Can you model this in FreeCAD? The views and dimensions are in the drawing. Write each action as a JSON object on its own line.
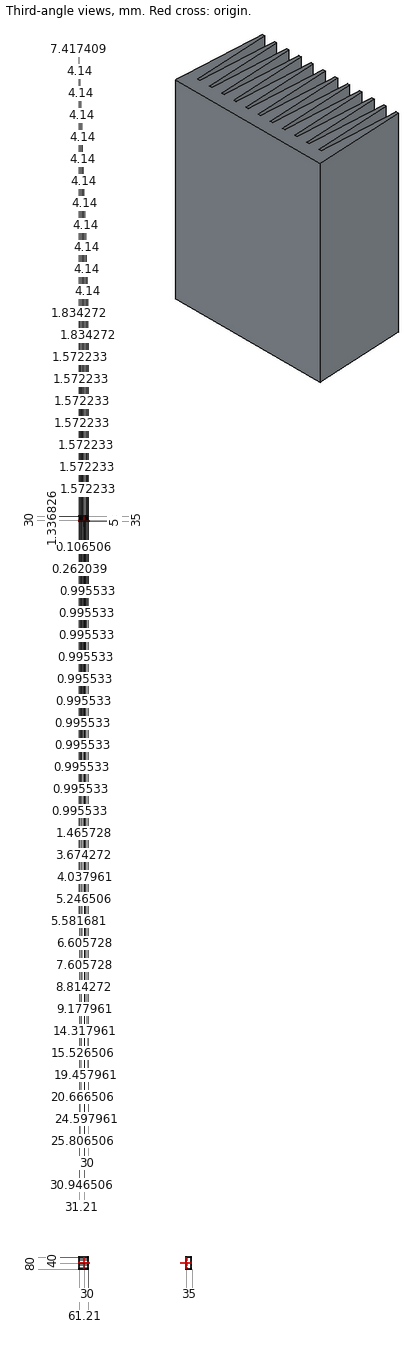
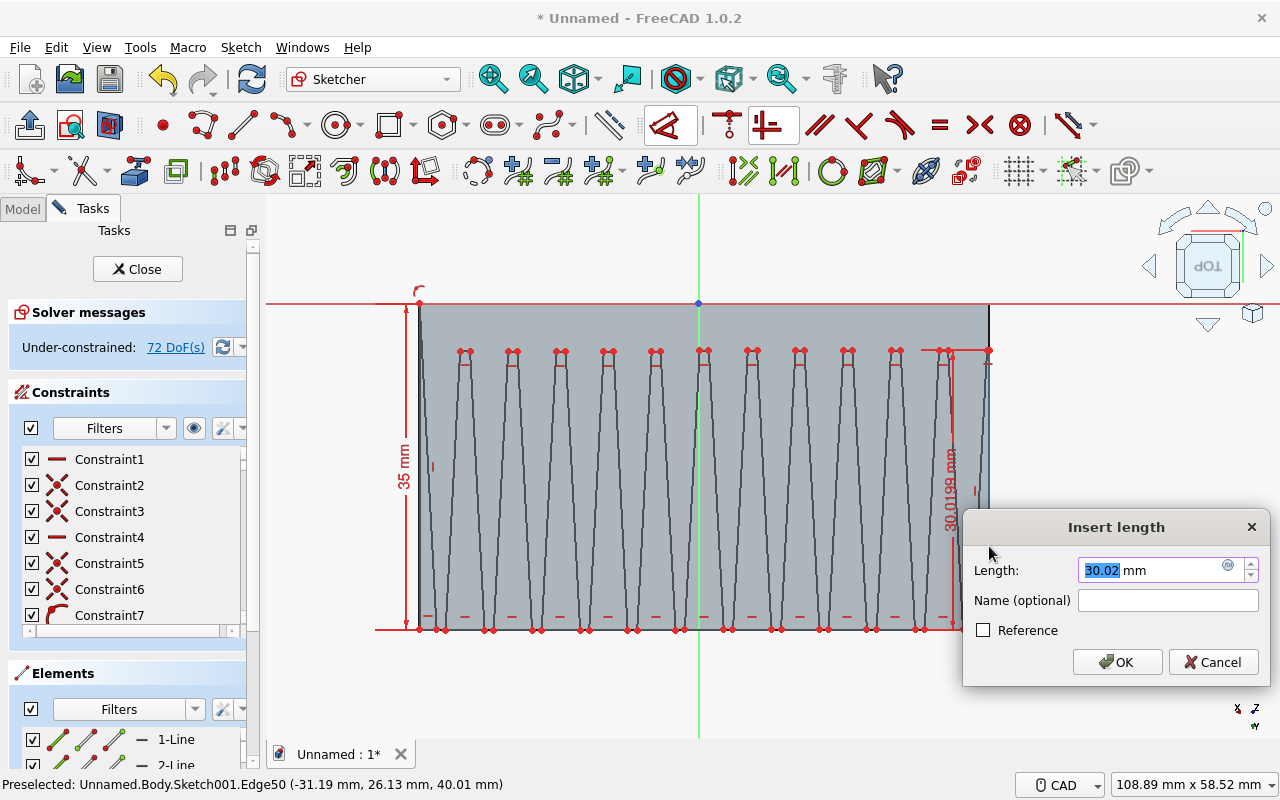
{"action": "type", "text": "30"}
{"action": "key", "text": "Return"}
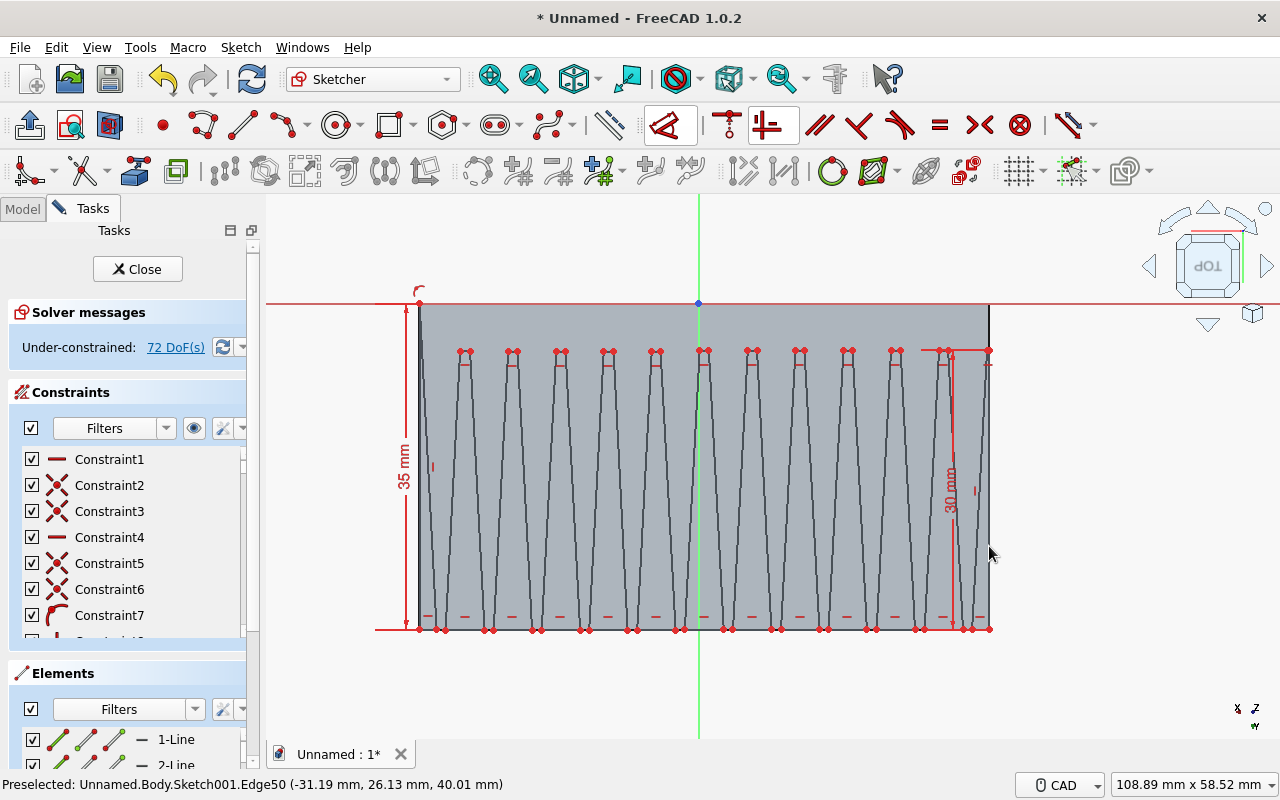
{"action": "scroll", "coordinate": [470, 351], "scroll_direction": "up", "scroll_amount": 2}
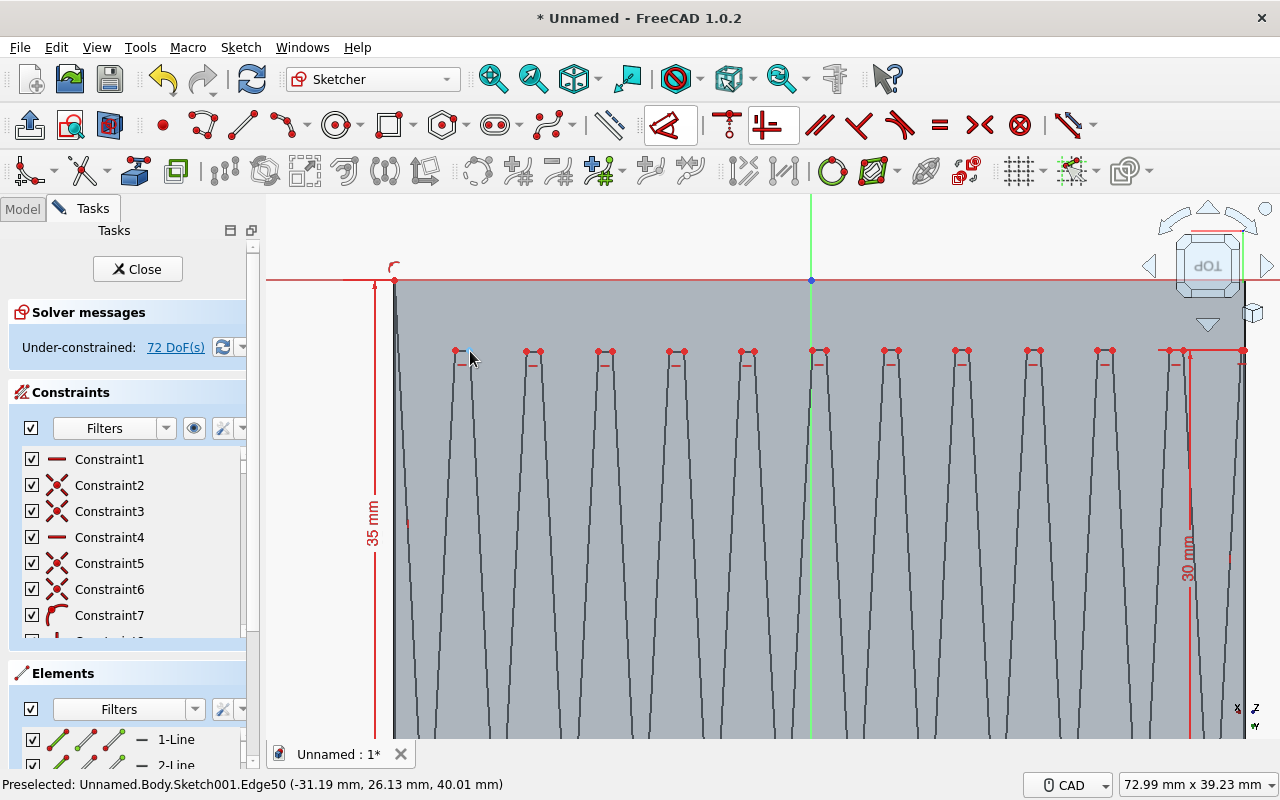
{"action": "left_click", "coordinate": [470, 351]}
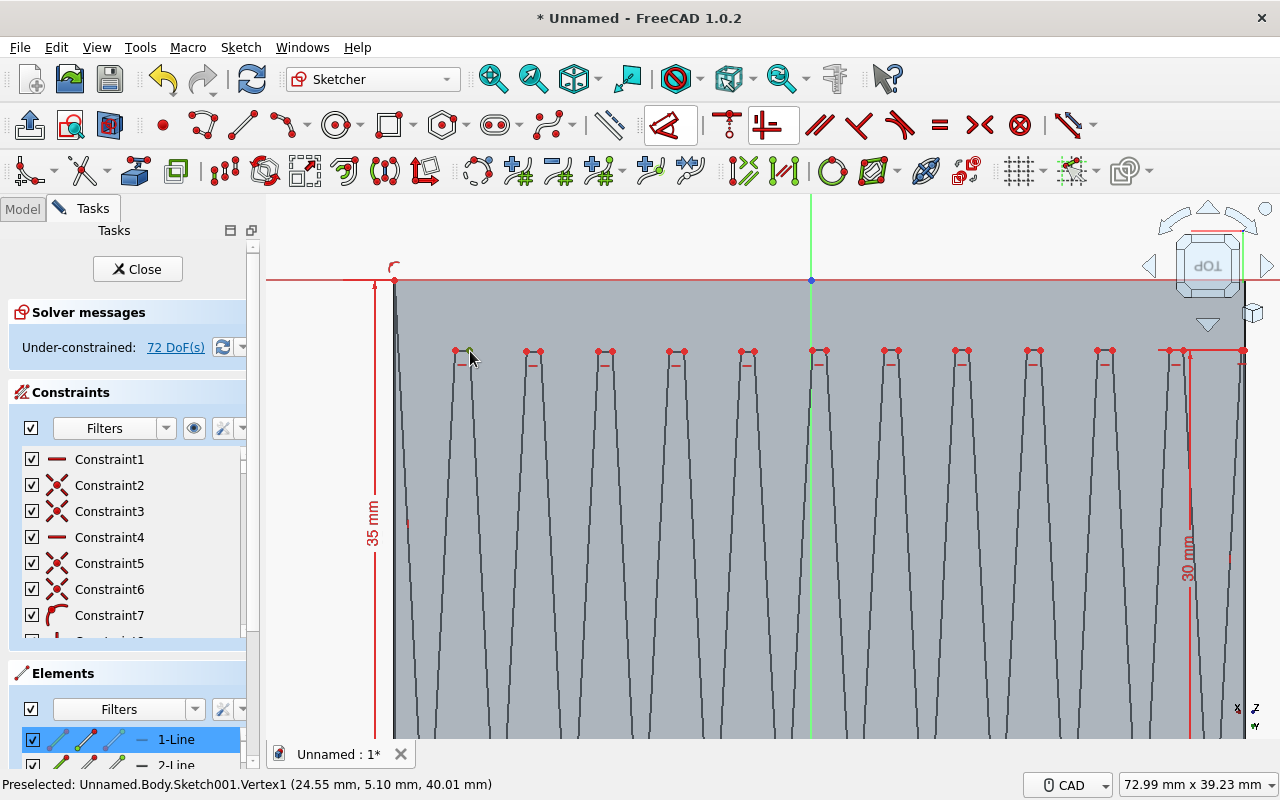
{"action": "left_click", "coordinate": [692, 126]}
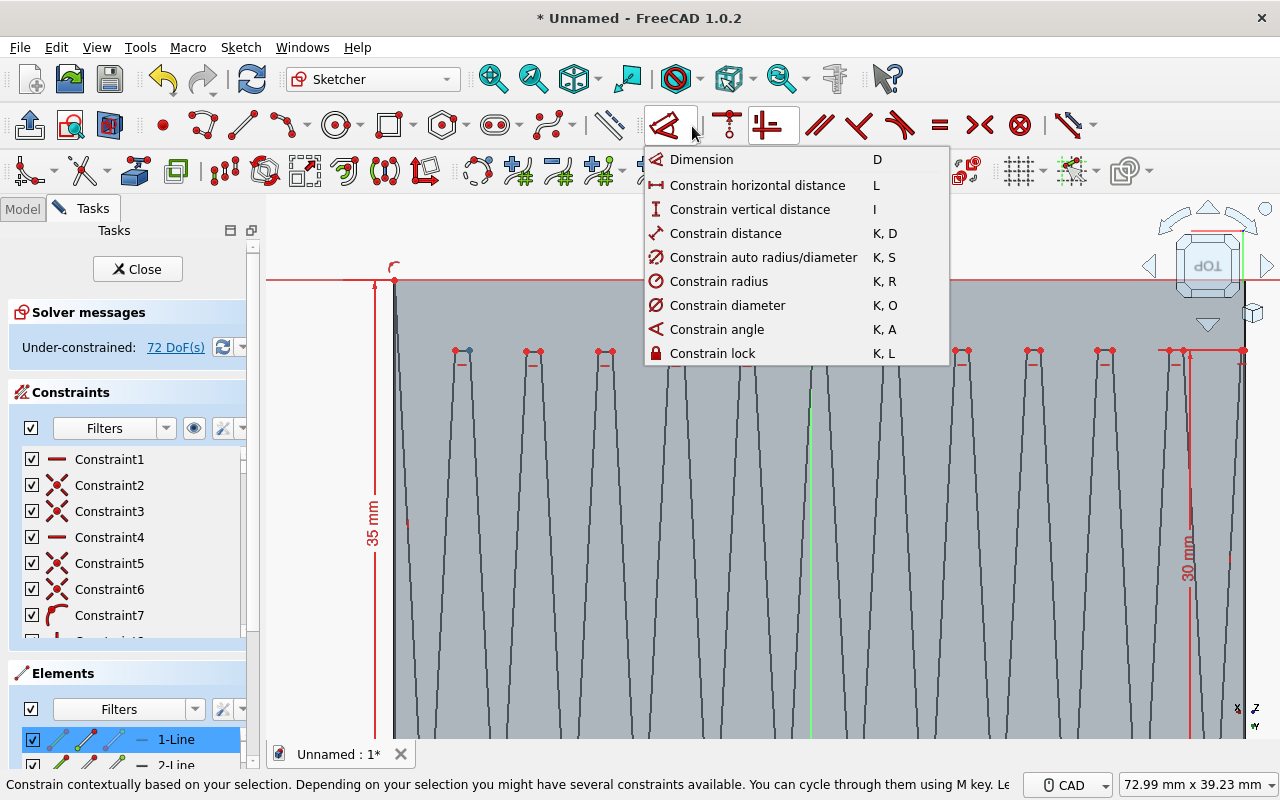
{"action": "left_click", "coordinate": [797, 209]}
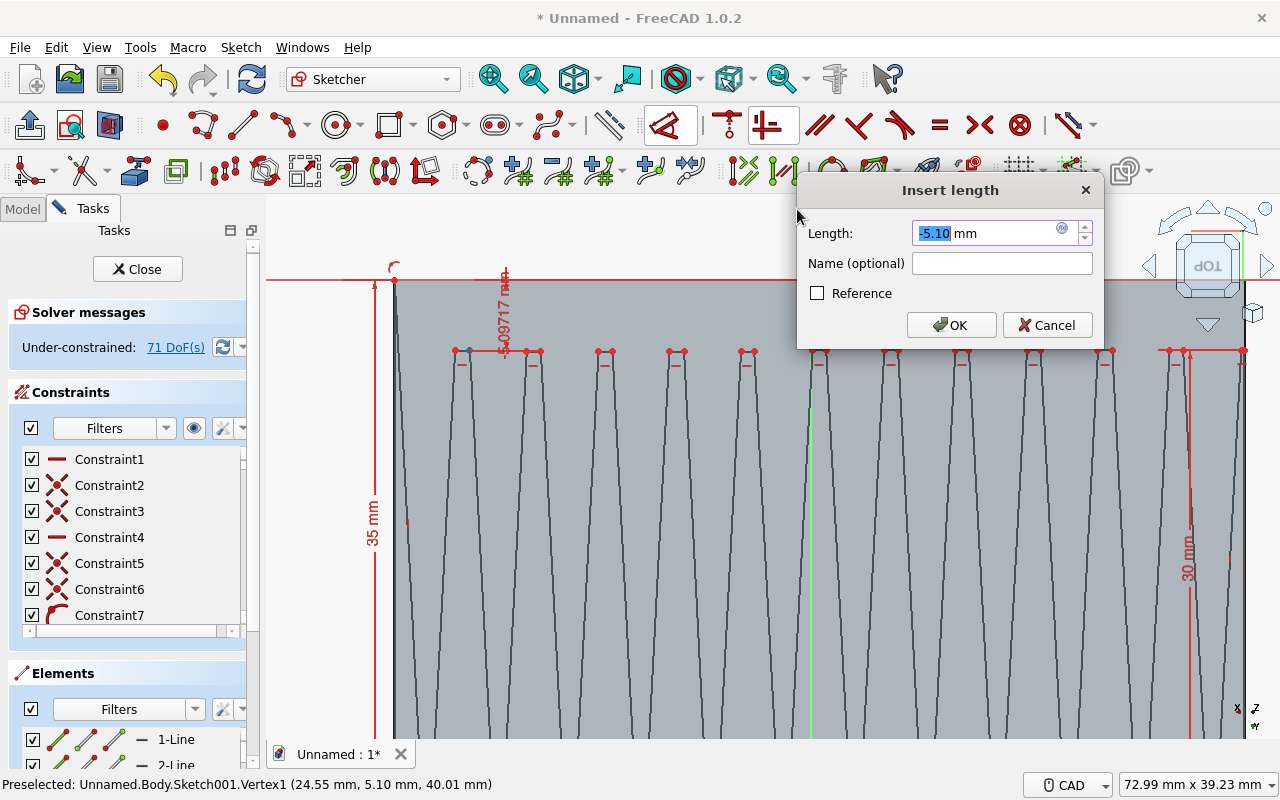
{"action": "type", "text": "-5"}
{"action": "key", "text": "Return"}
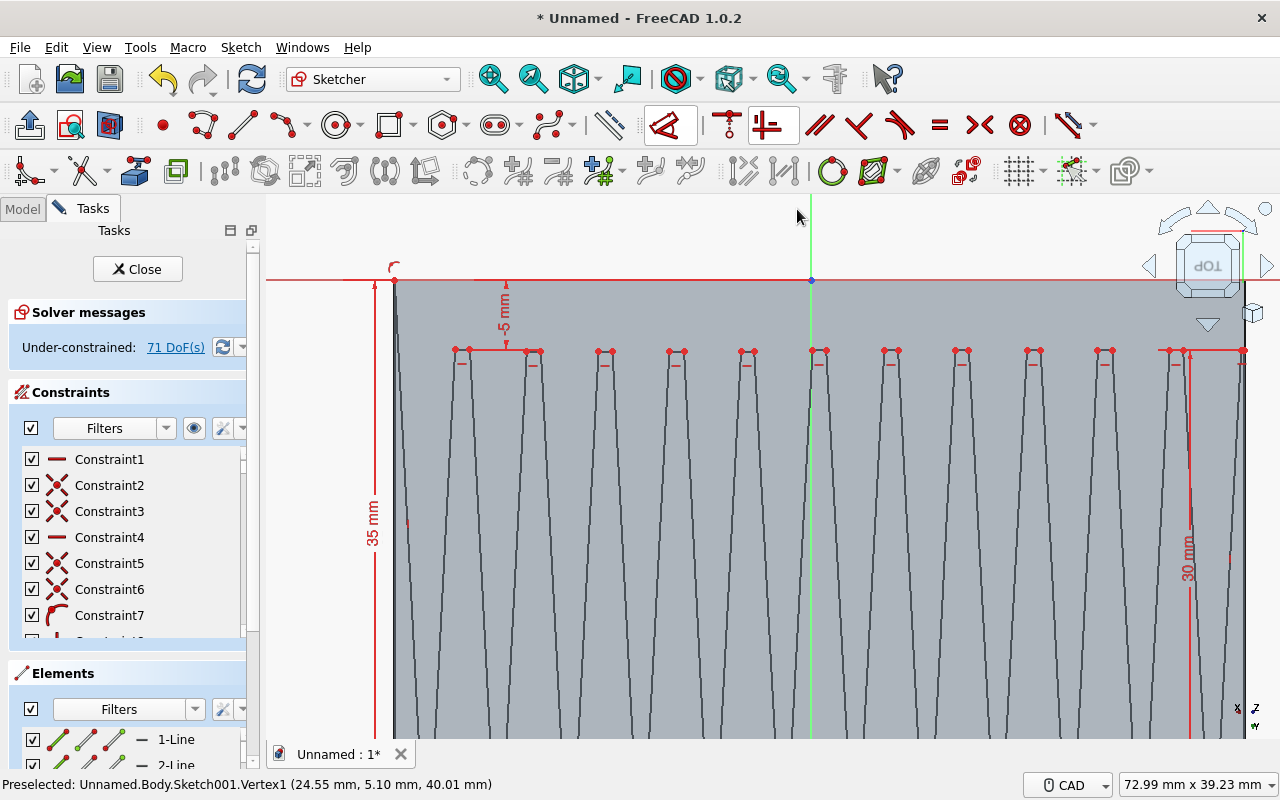
{"action": "left_click", "coordinate": [541, 352]}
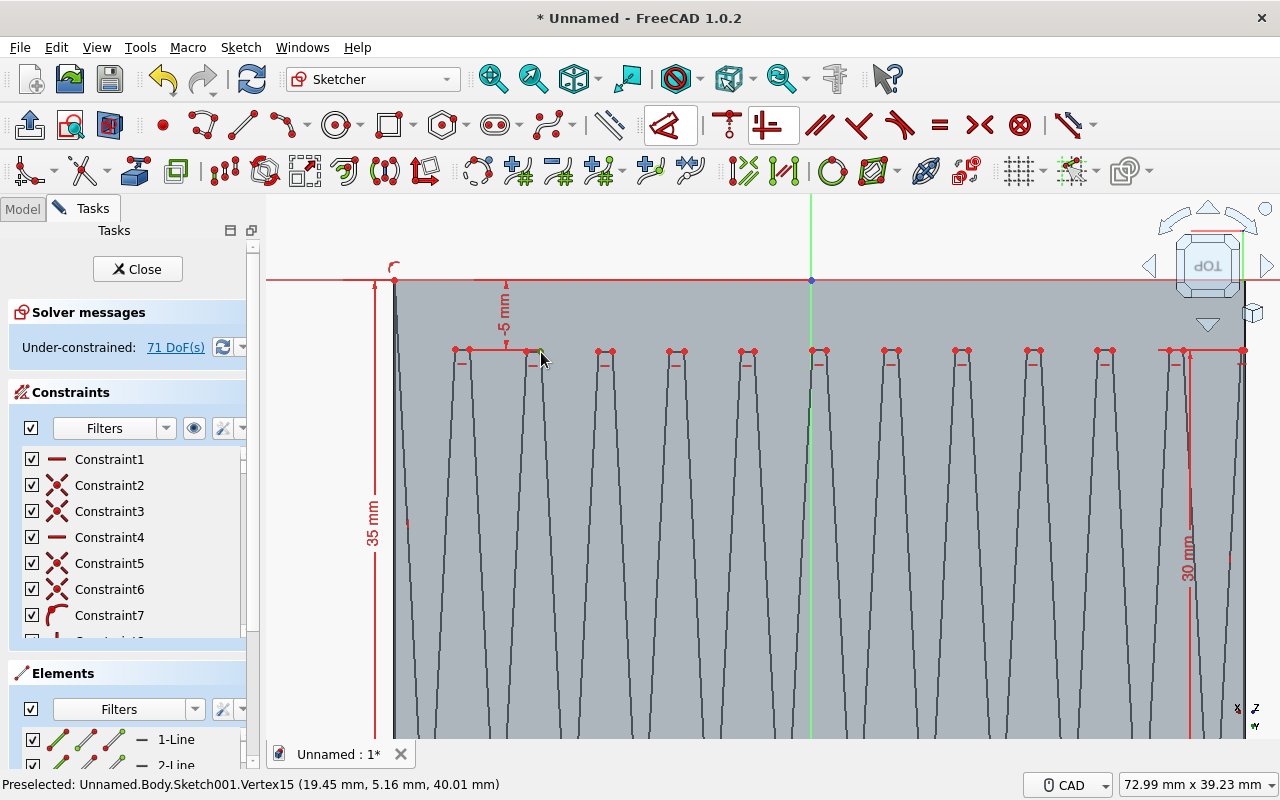
{"action": "key", "text": "i"}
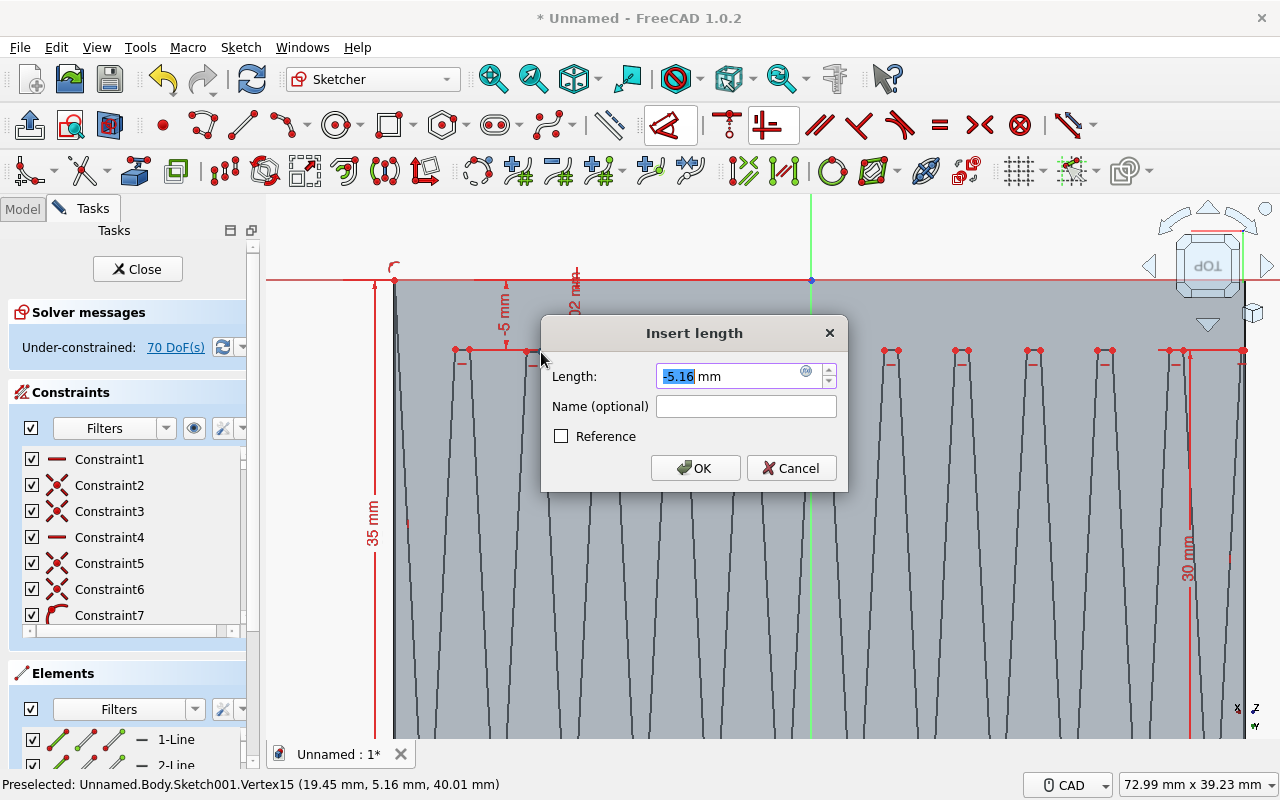
{"action": "type", "text": "-5"}
{"action": "key", "text": "Return"}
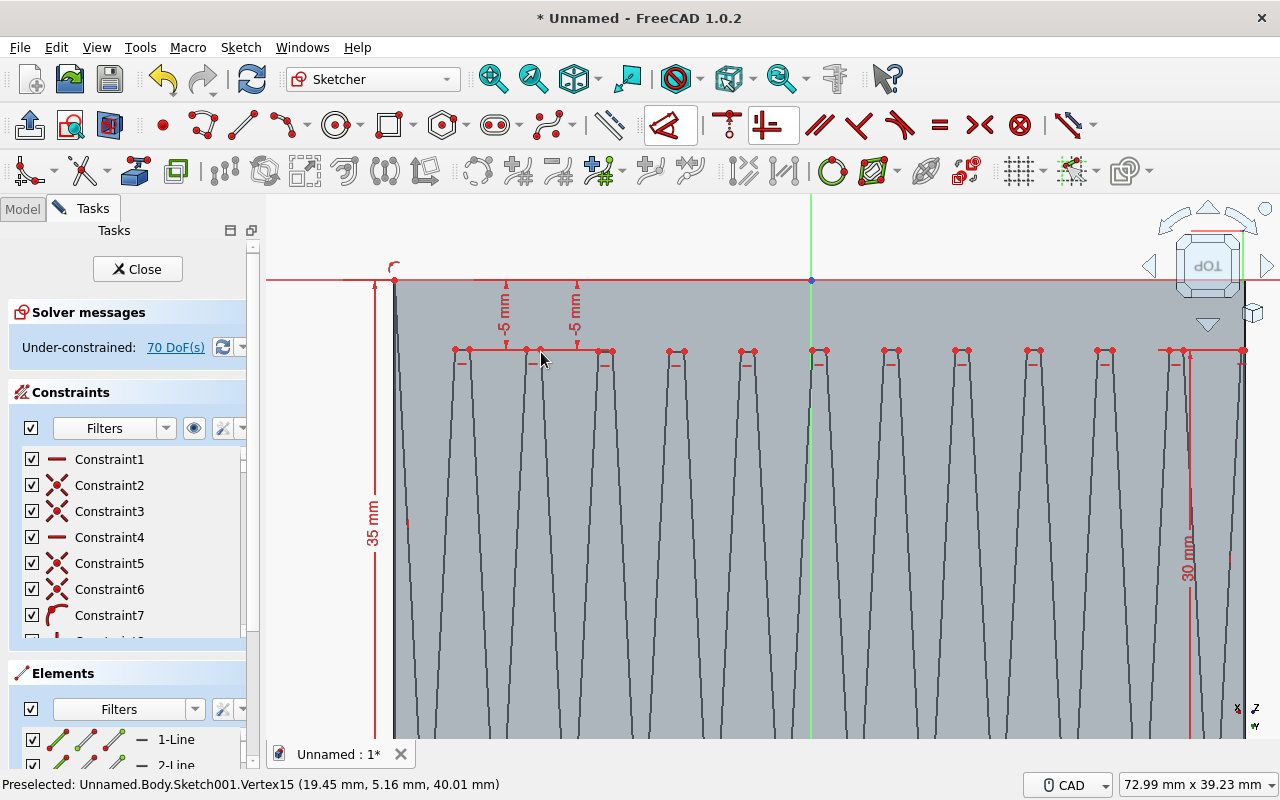
{"action": "left_click", "coordinate": [612, 352]}